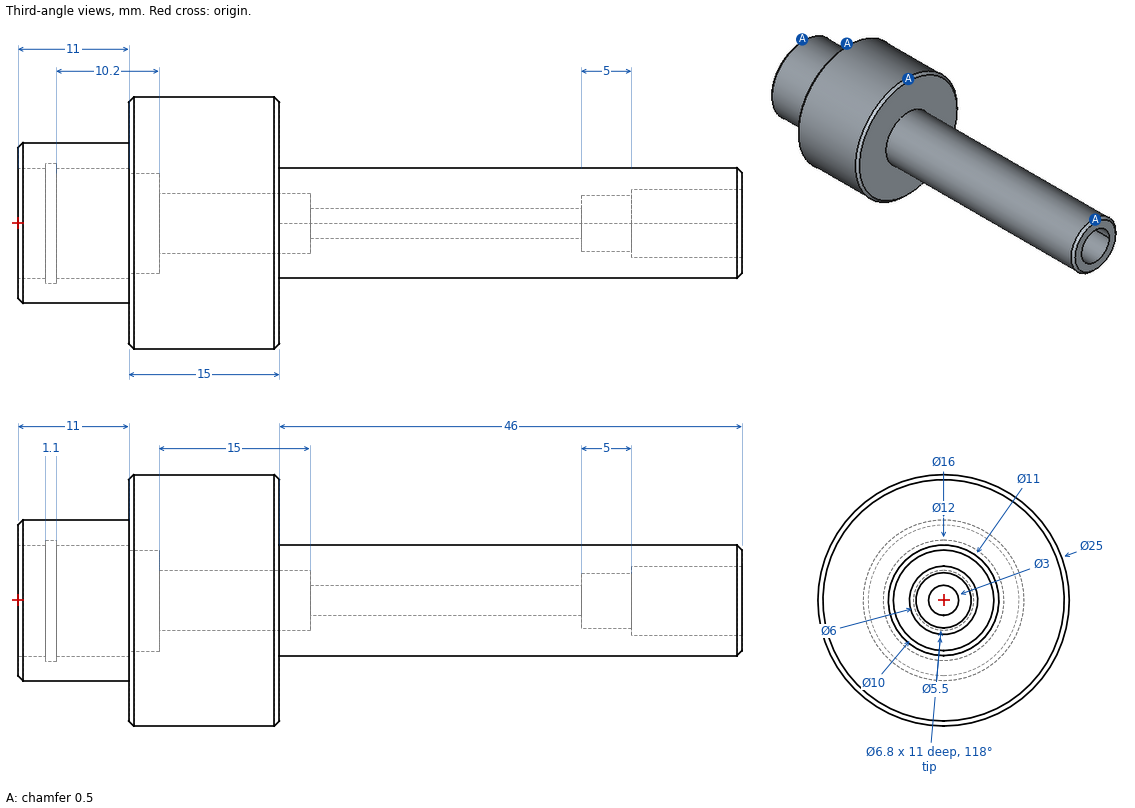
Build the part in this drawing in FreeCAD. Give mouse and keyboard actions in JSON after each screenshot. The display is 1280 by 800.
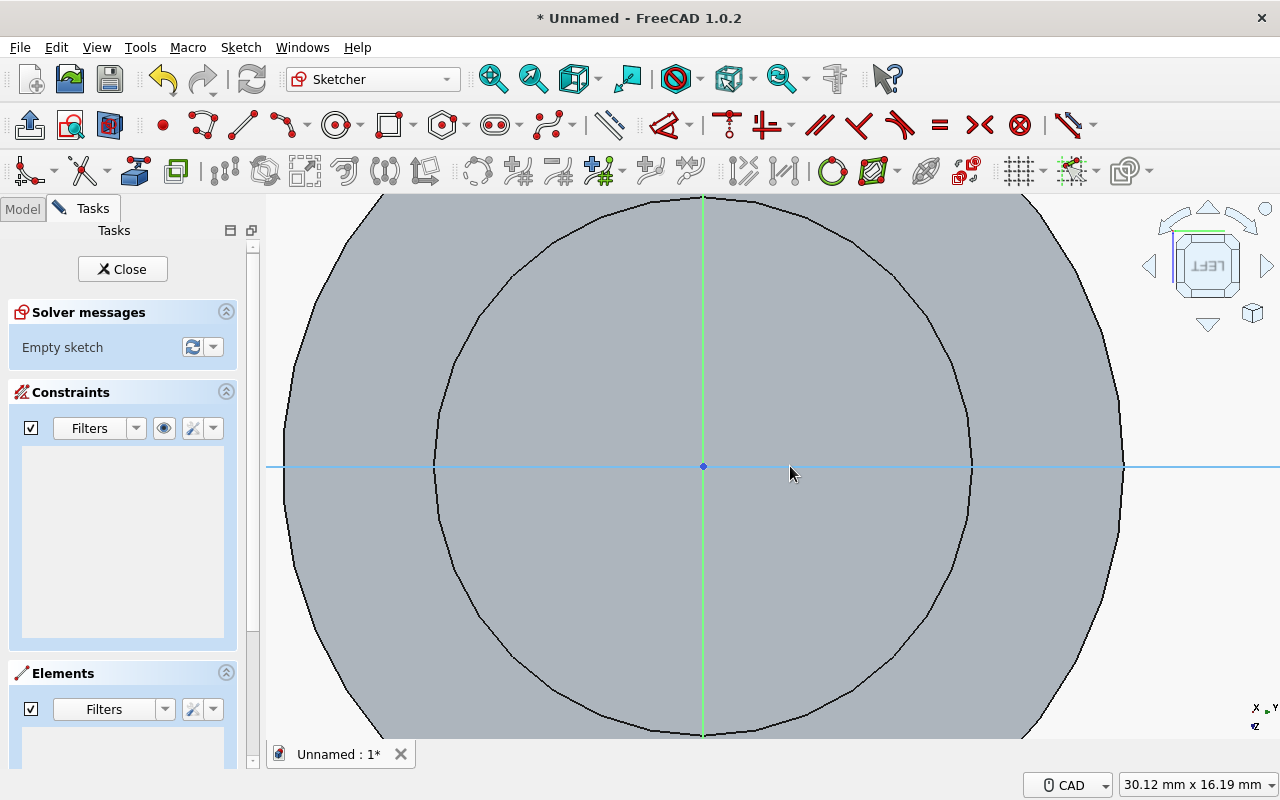
{"action": "key", "text": "g c"}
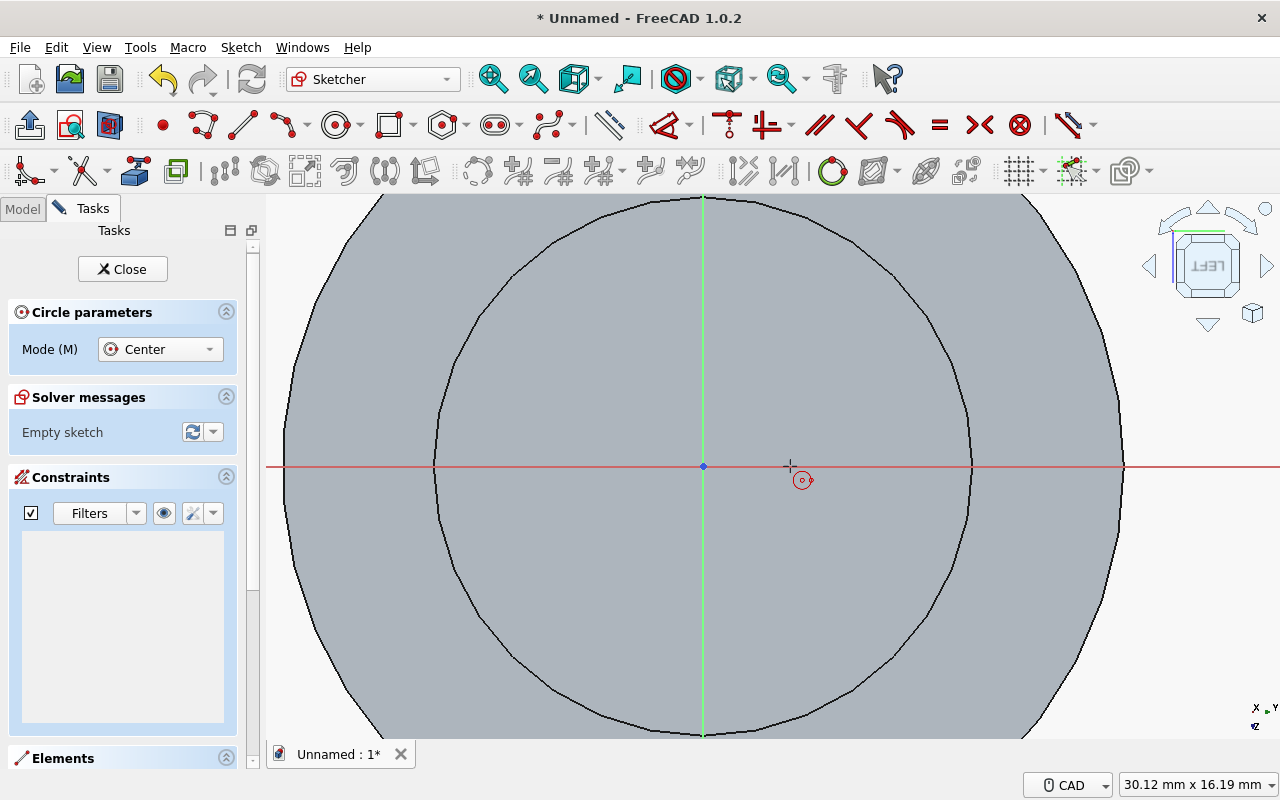
{"action": "left_click", "coordinate": [703, 466]}
{"action": "mouse_move", "coordinate": [834, 336]}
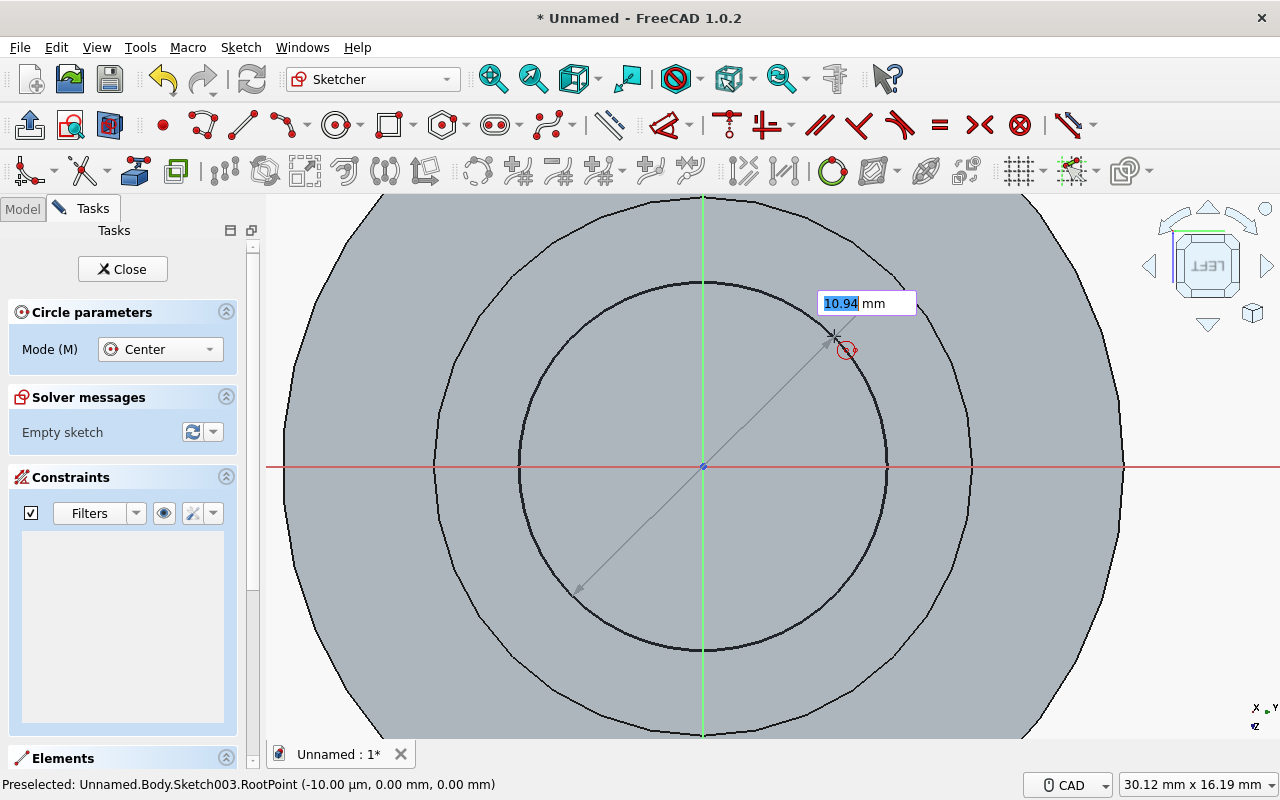
{"action": "type", "text": "11"}
{"action": "key", "text": "Return"}
{"action": "key", "text": "Escape"}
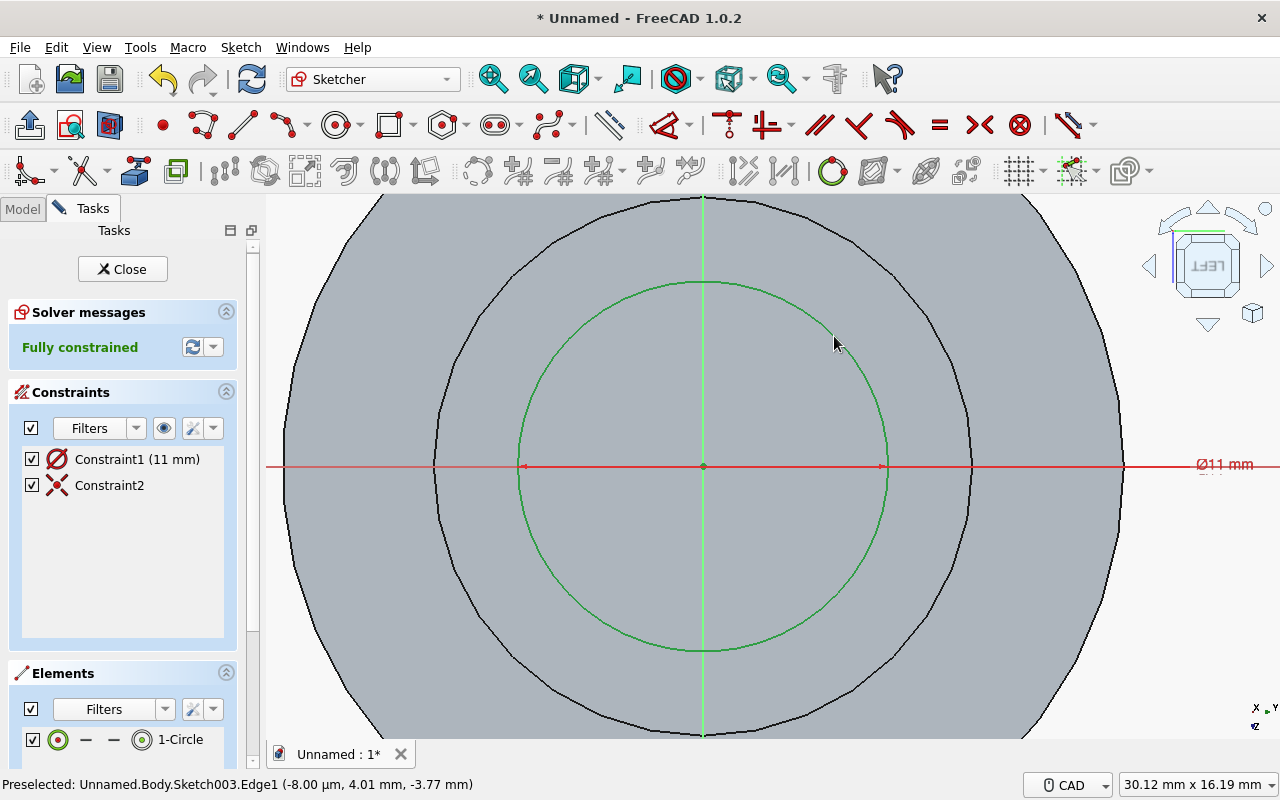
{"action": "left_click", "coordinate": [123, 269]}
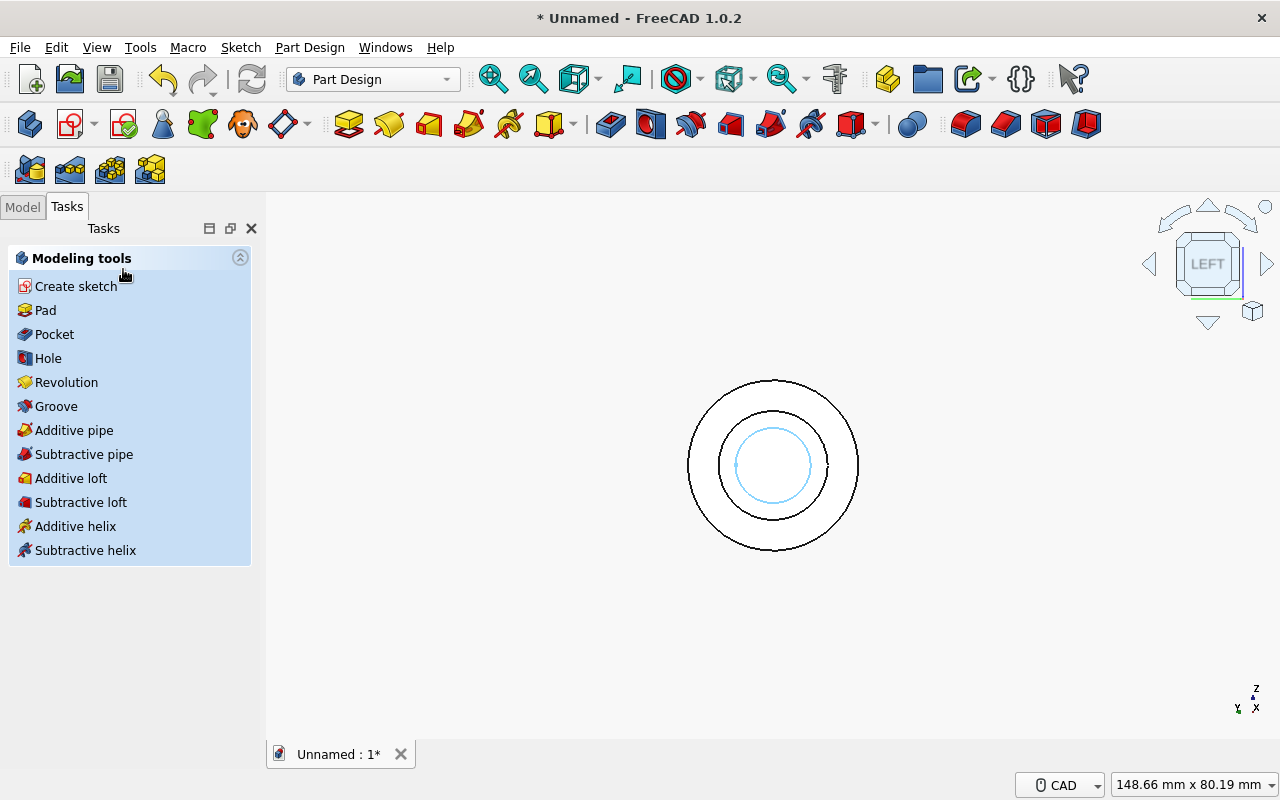
{"action": "left_click", "coordinate": [612, 124]}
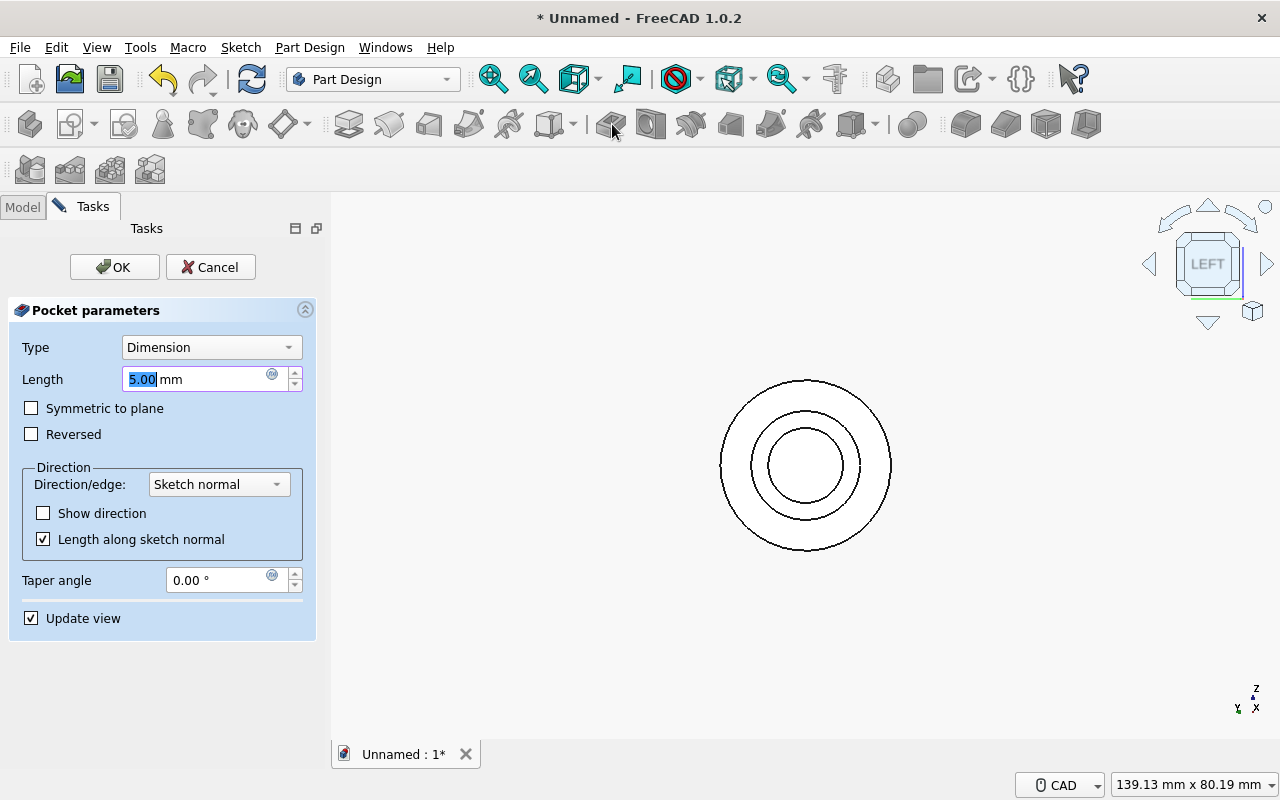
{"action": "type", "text": "11"}
{"action": "key", "text": "Tab"}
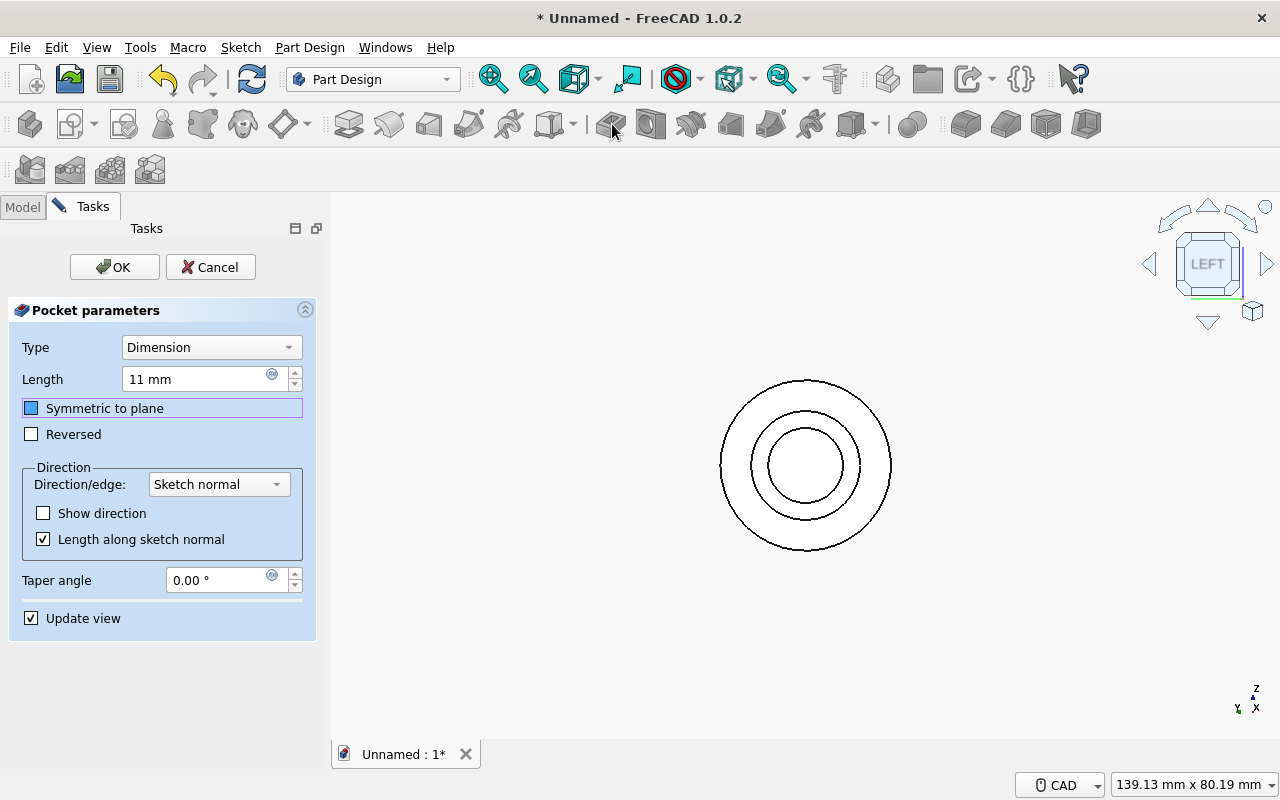
{"action": "left_click", "coordinate": [115, 267]}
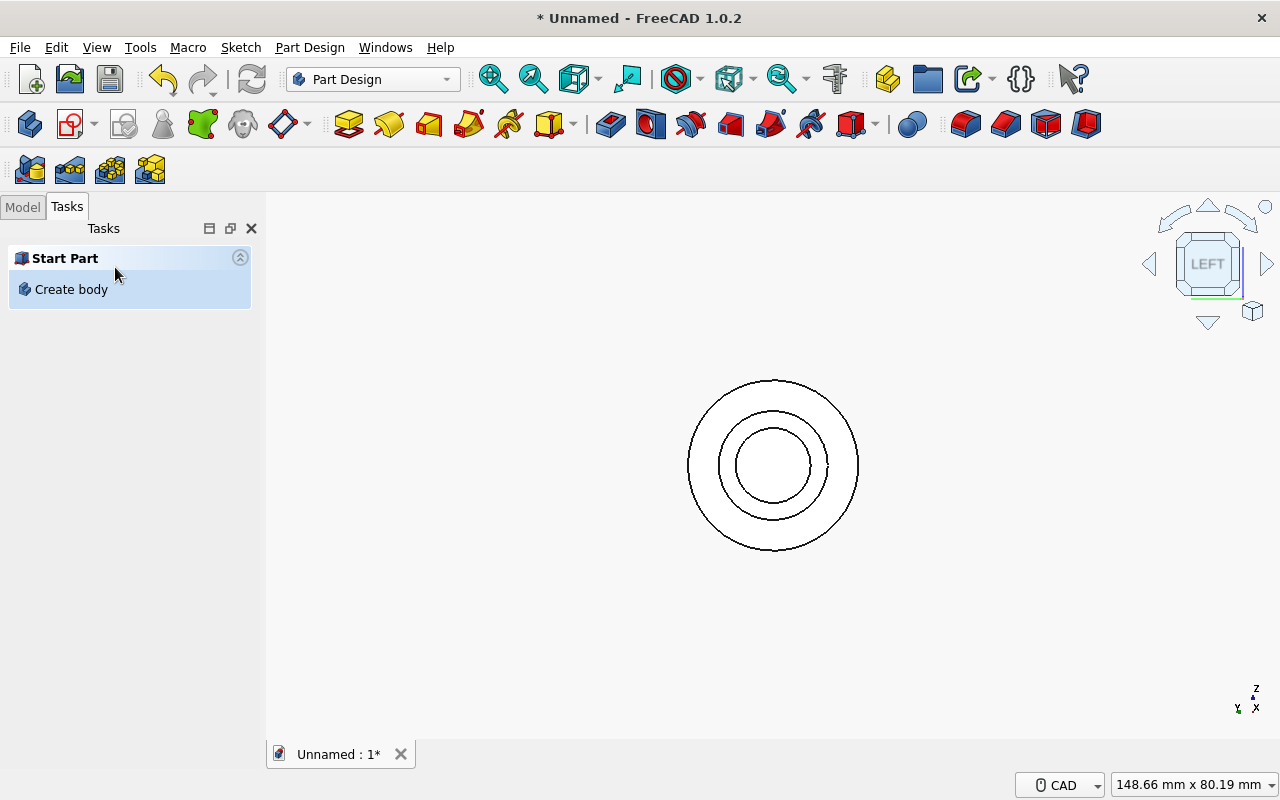
{"action": "left_click", "coordinate": [494, 80]}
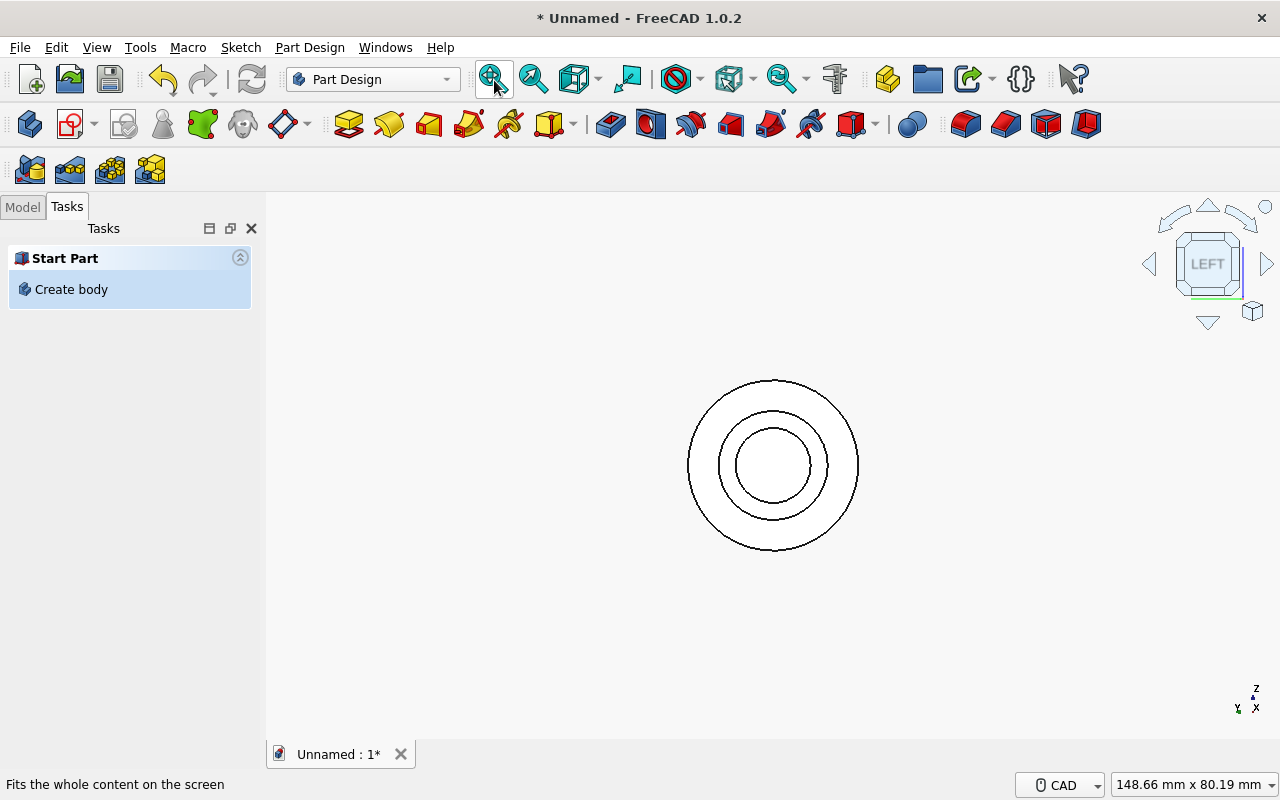
{"action": "left_click", "coordinate": [23, 206]}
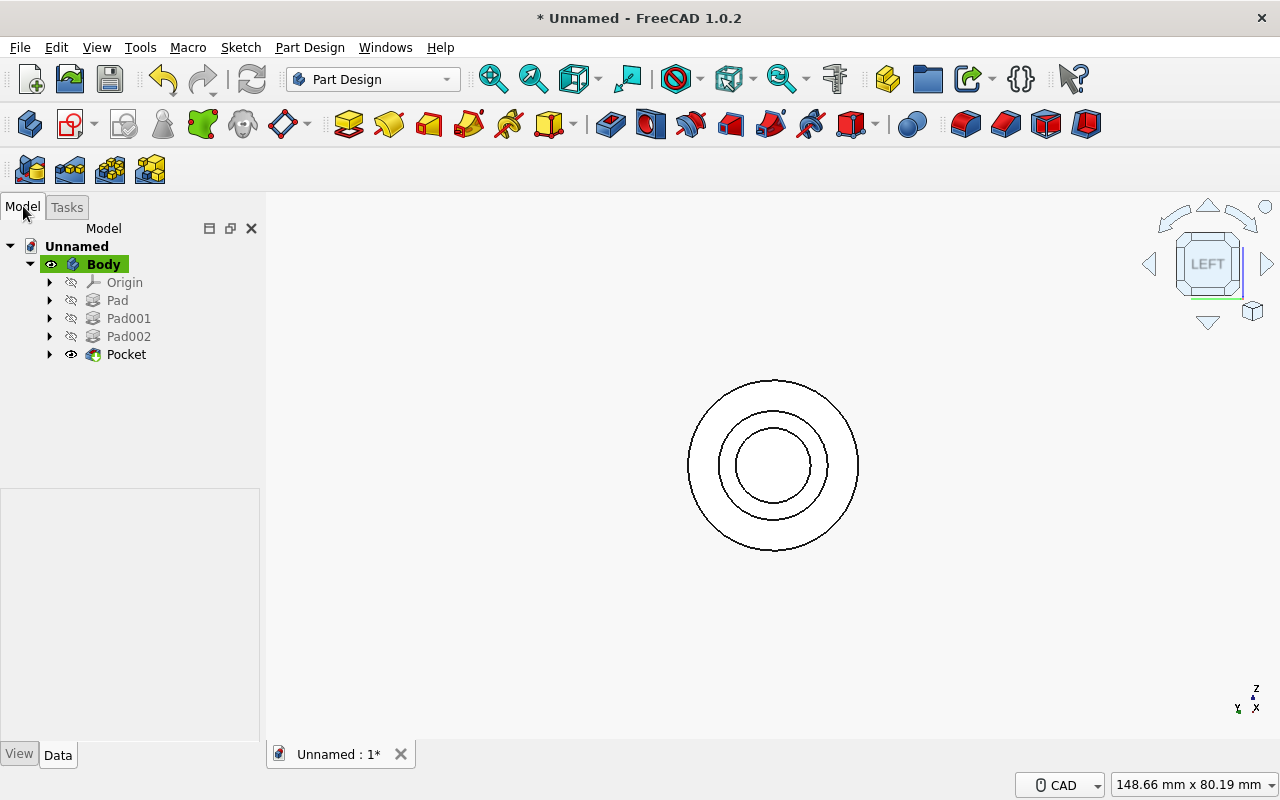
{"action": "left_click", "coordinate": [50, 282]}